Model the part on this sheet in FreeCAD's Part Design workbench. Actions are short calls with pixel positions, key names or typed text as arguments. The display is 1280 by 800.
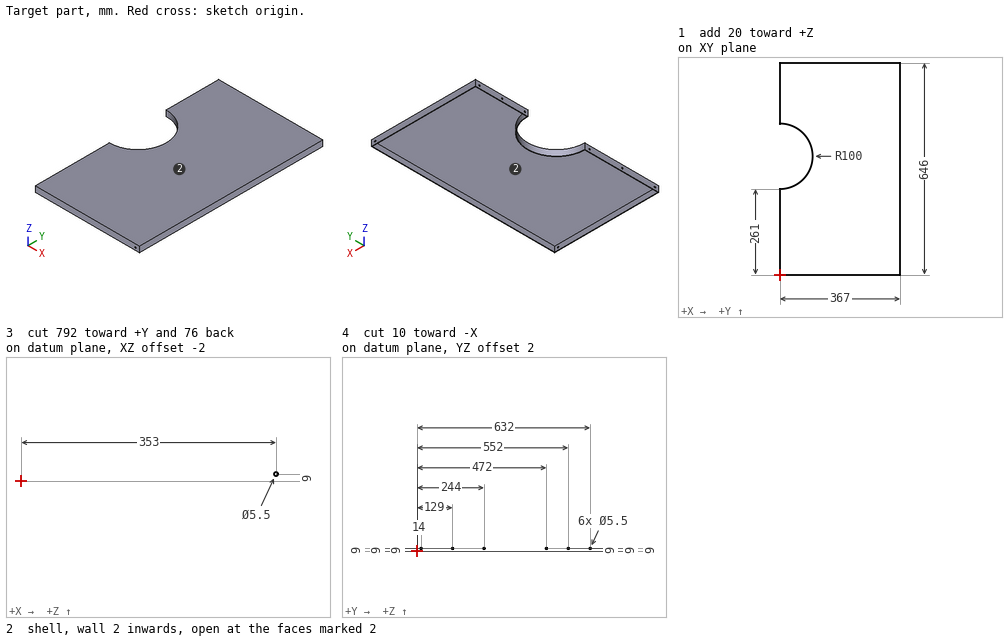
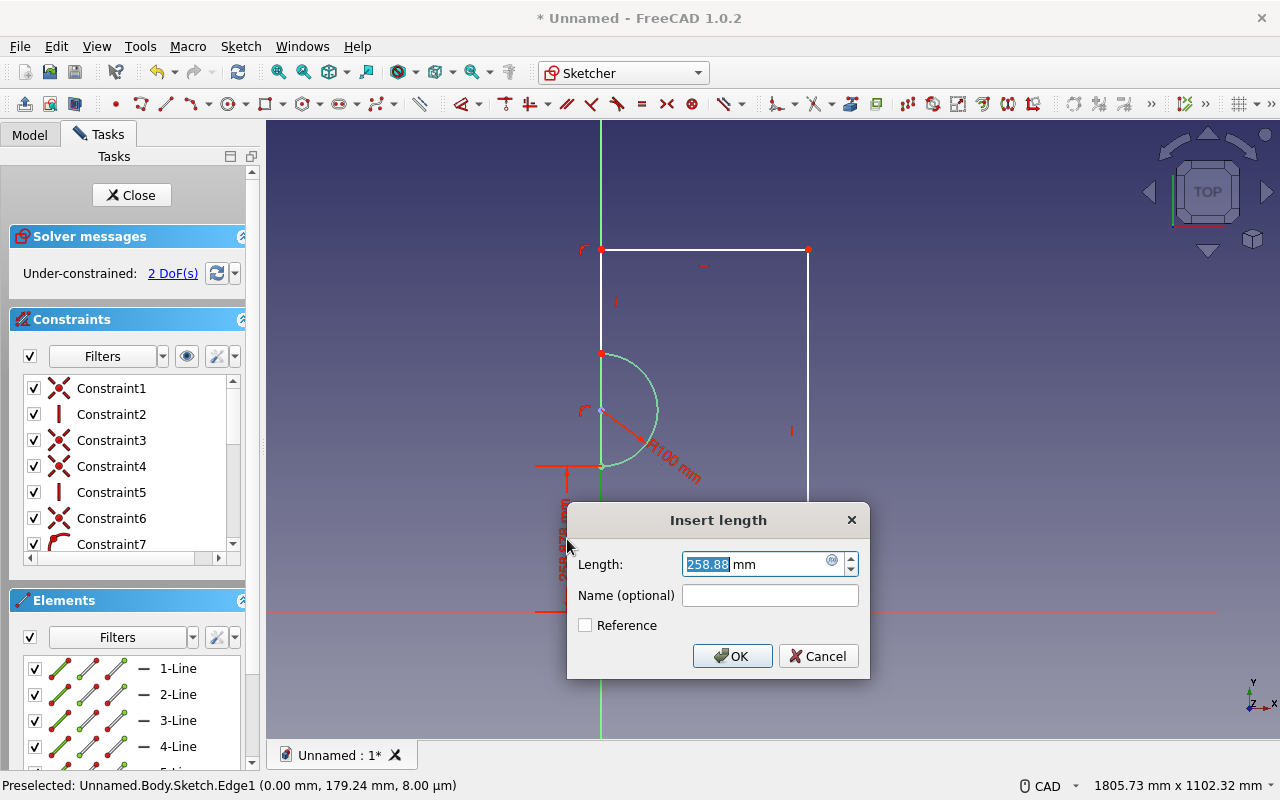
text(261)
key(Return)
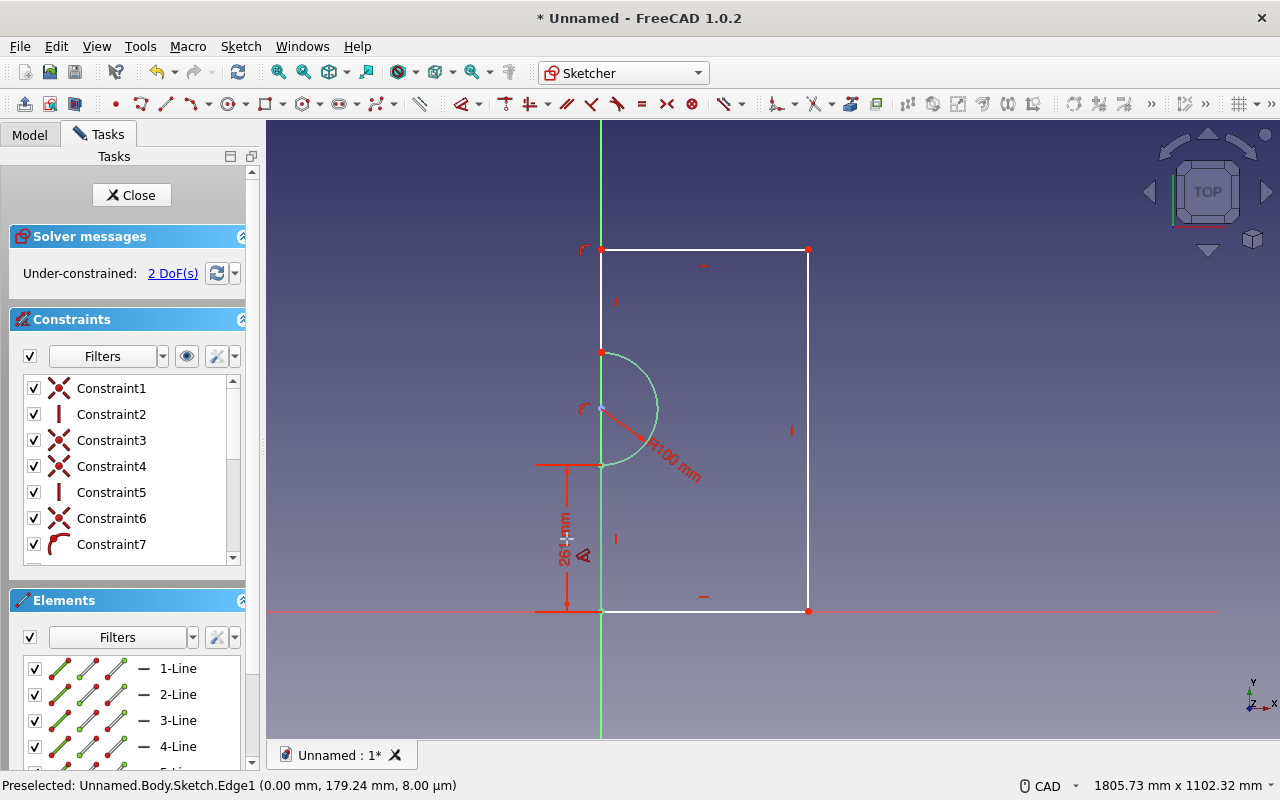
click(663, 612)
click(705, 646)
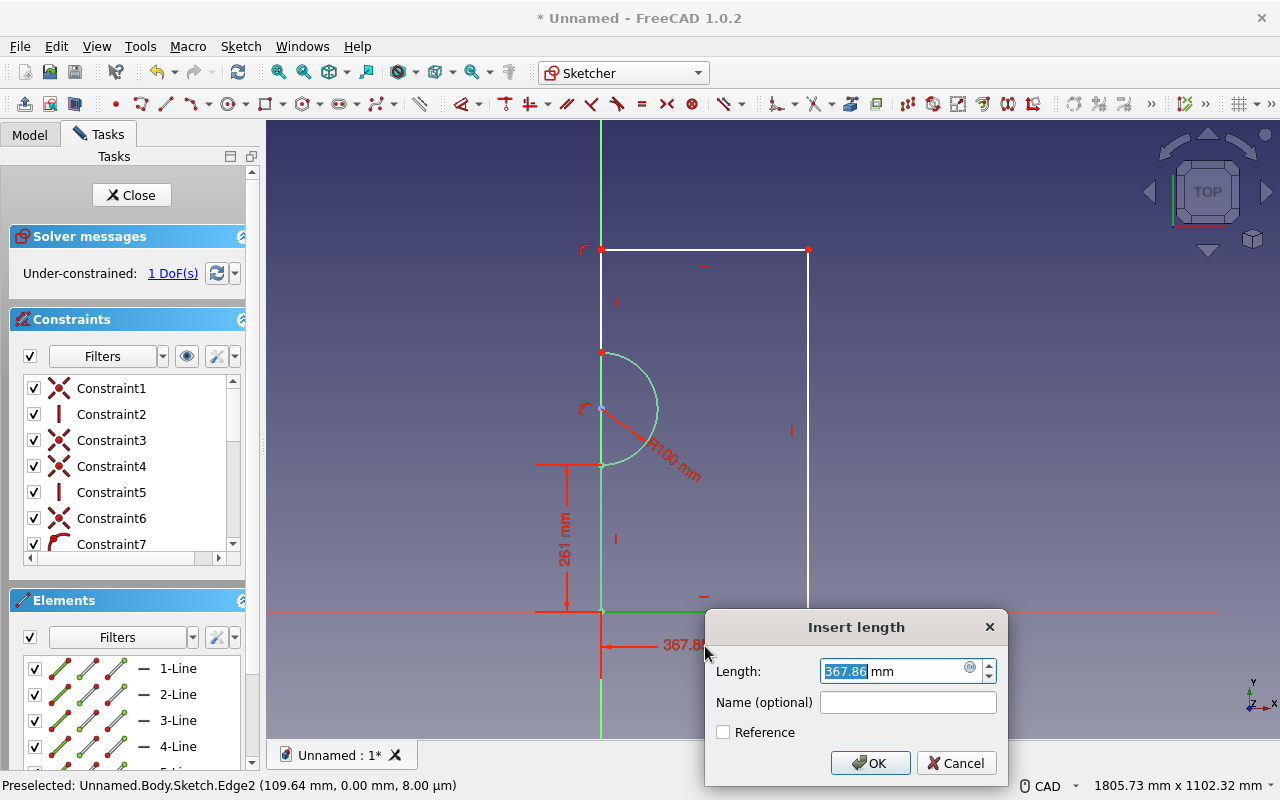
text(367)
key(Return)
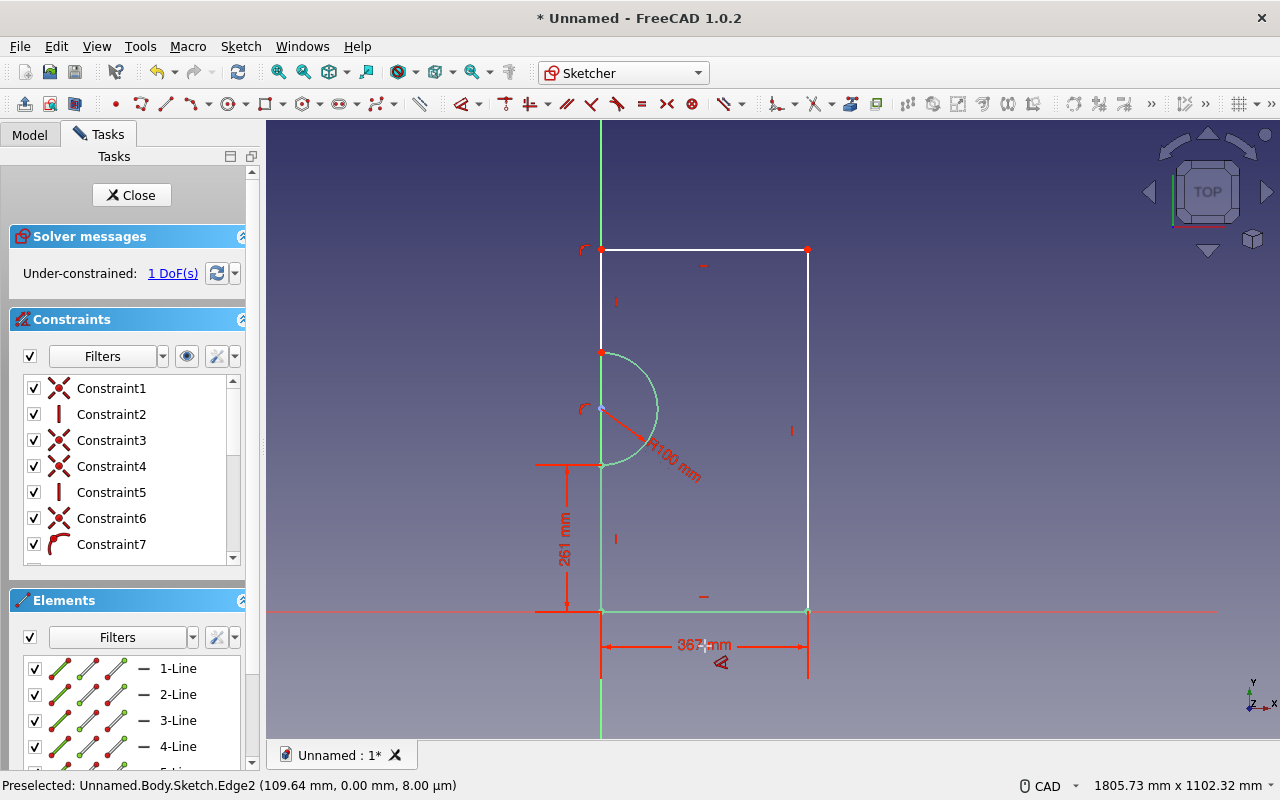
click(808, 503)
click(842, 431)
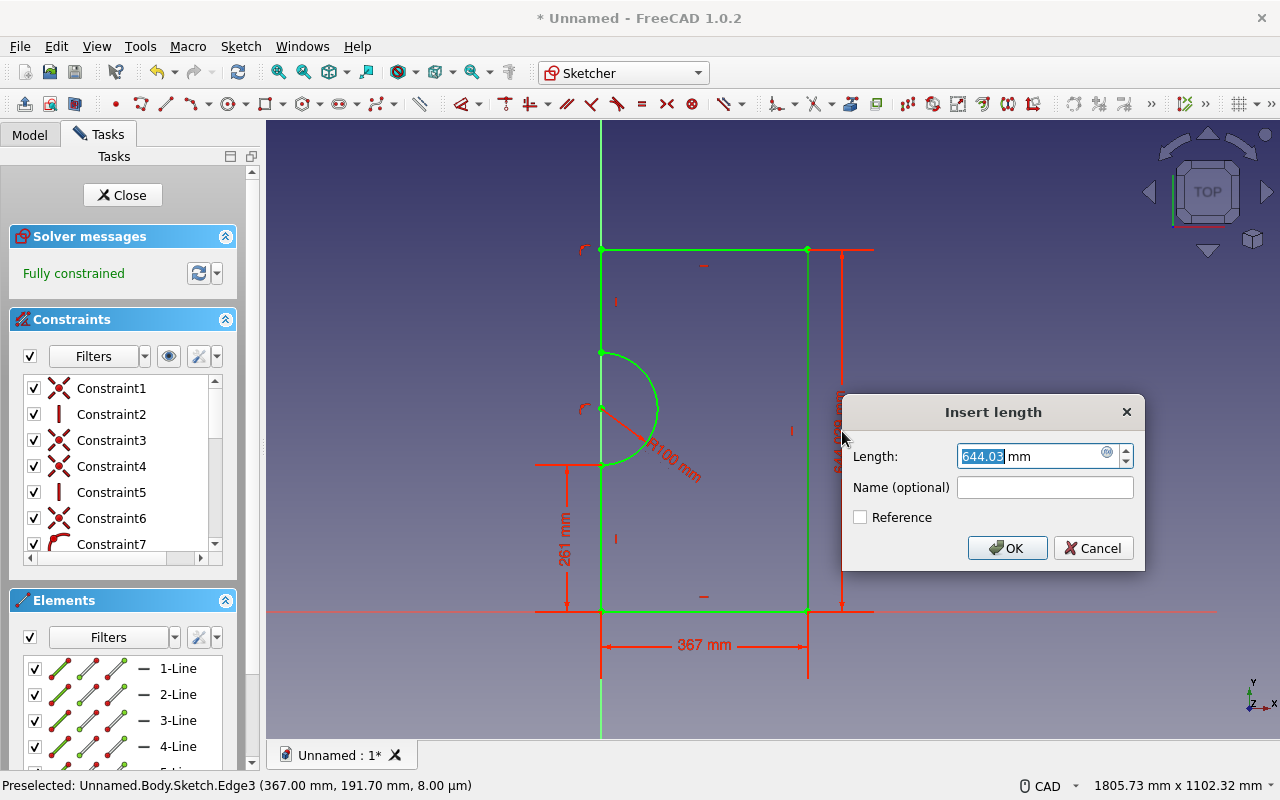
text(646)
key(Return)
key(Escape)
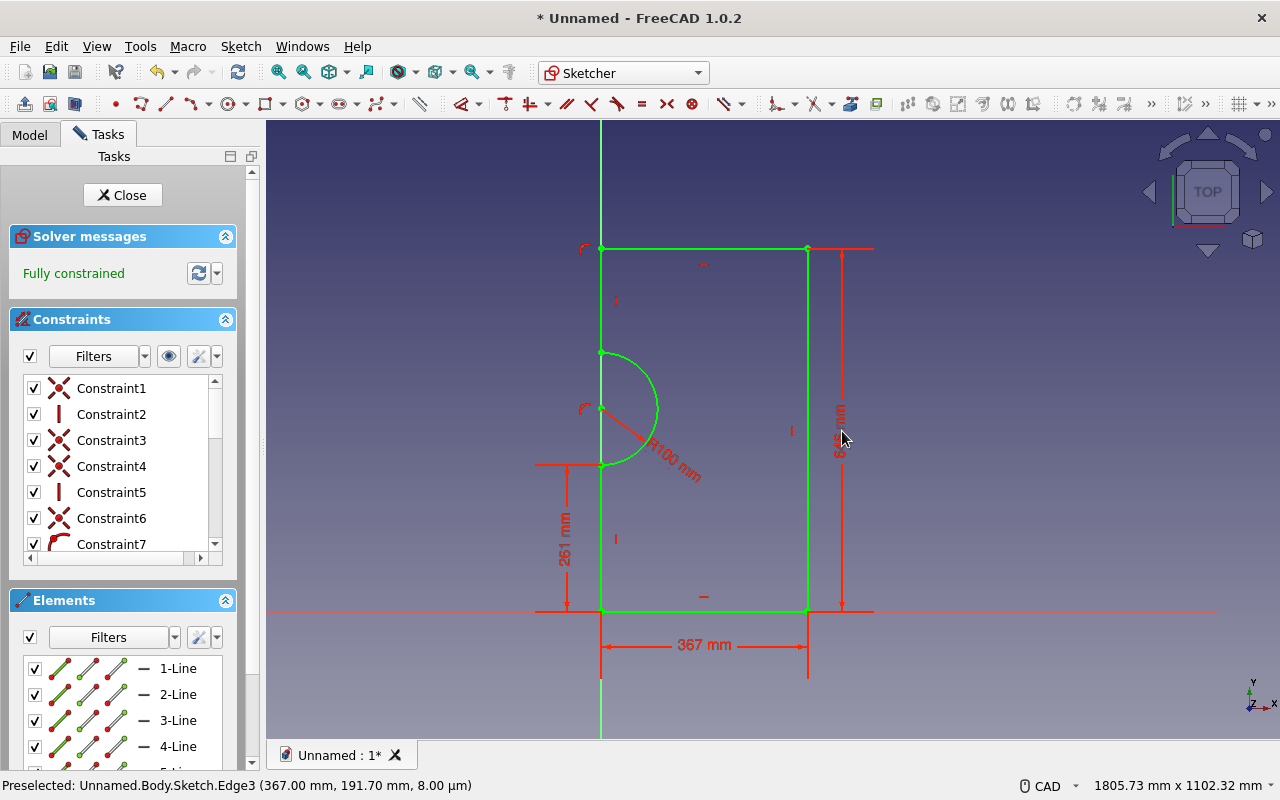
click(123, 195)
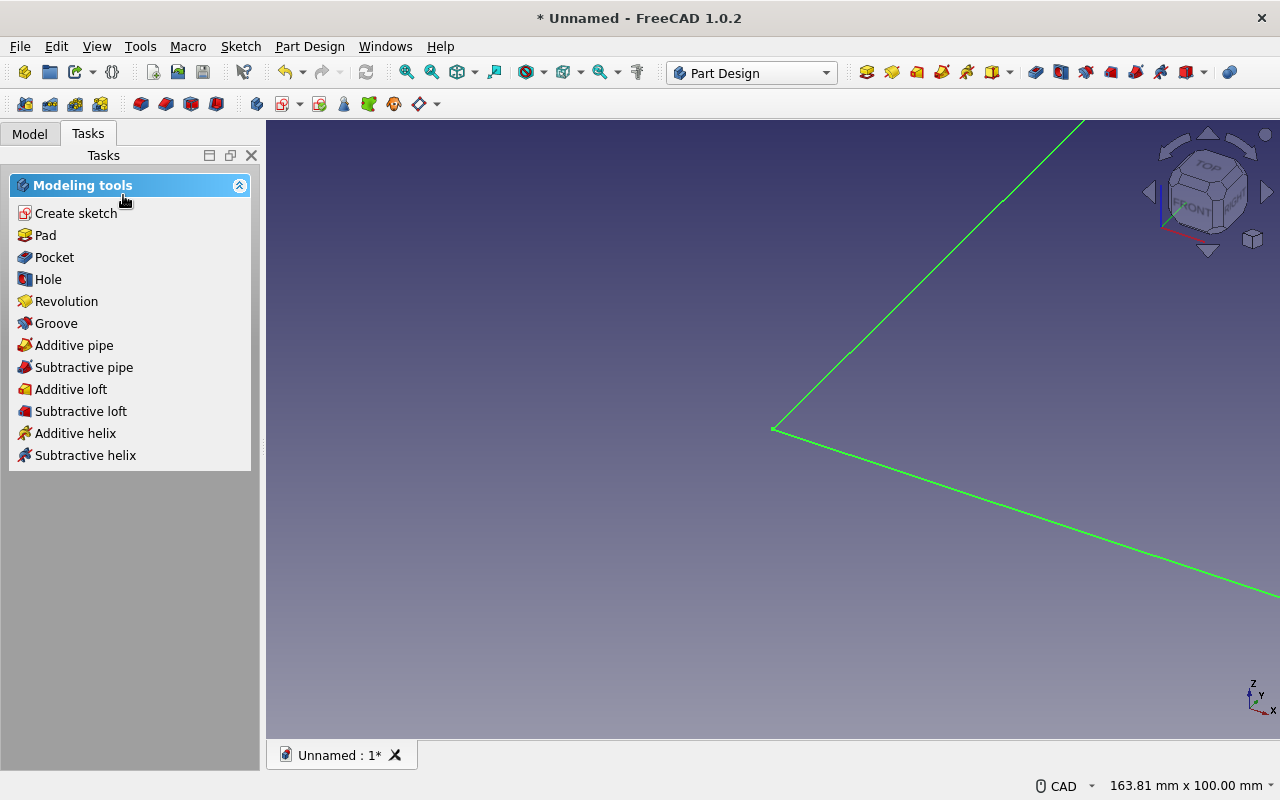
click(867, 72)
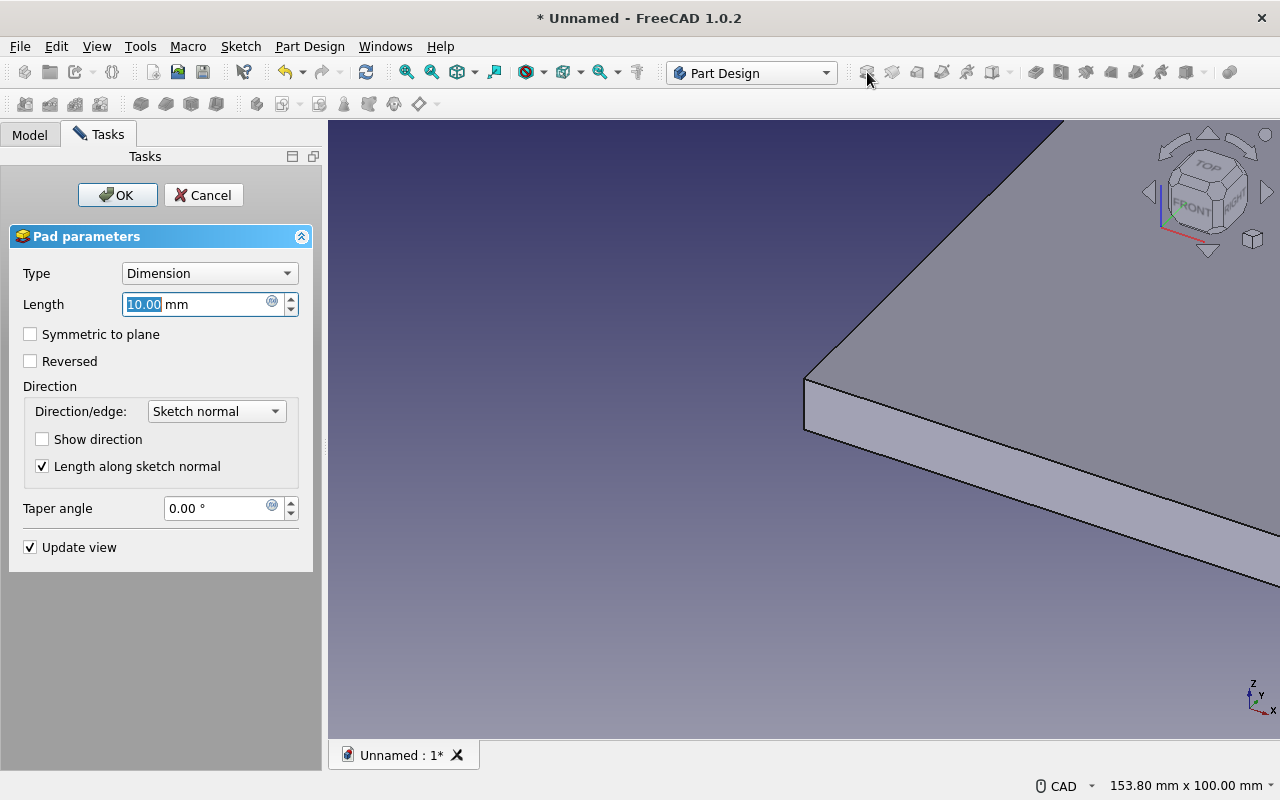
text(20)
key(Tab)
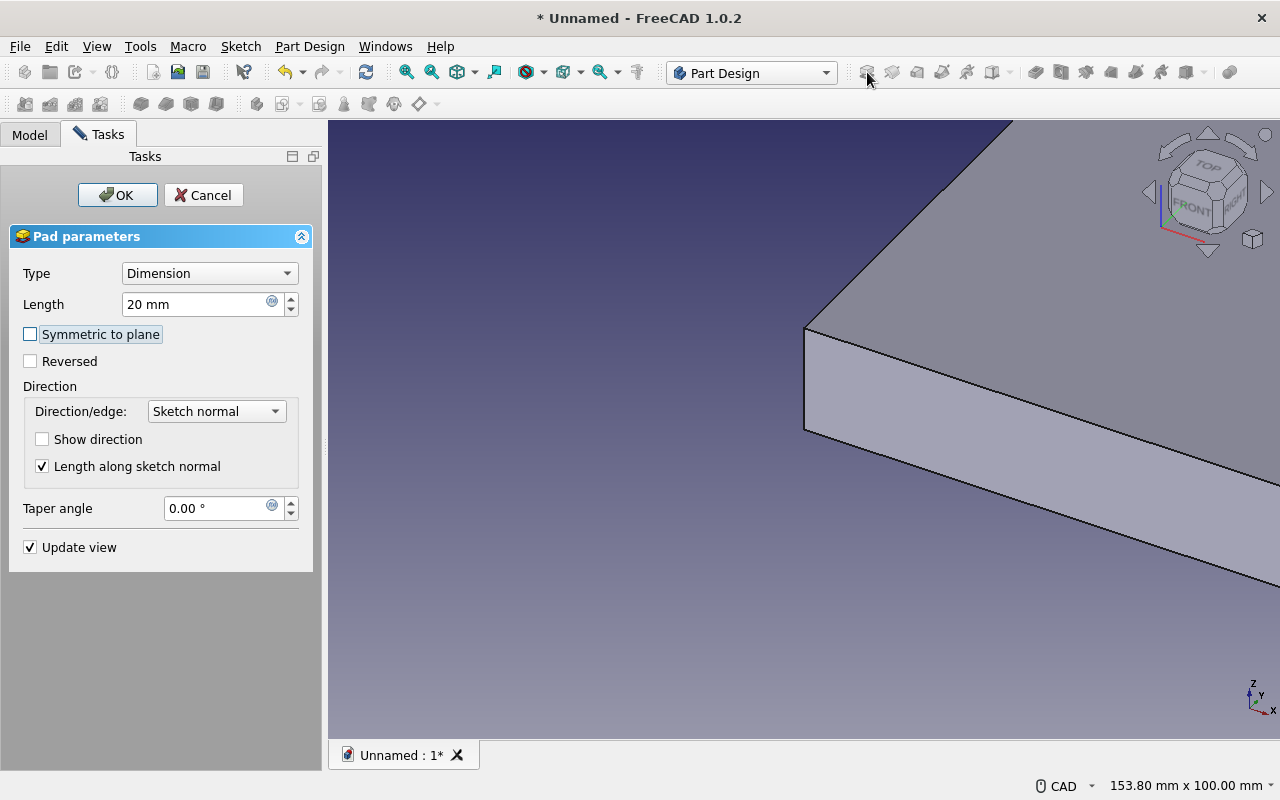
click(118, 195)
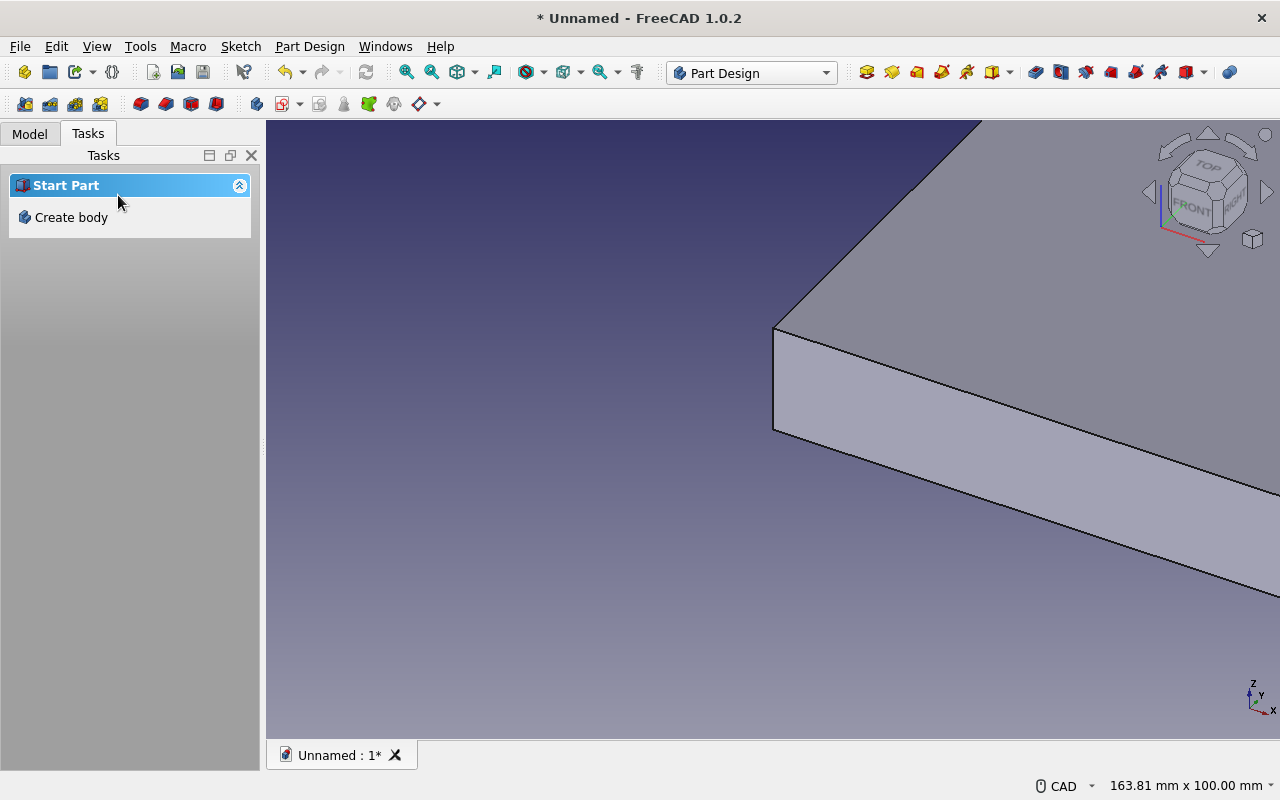
click(407, 72)